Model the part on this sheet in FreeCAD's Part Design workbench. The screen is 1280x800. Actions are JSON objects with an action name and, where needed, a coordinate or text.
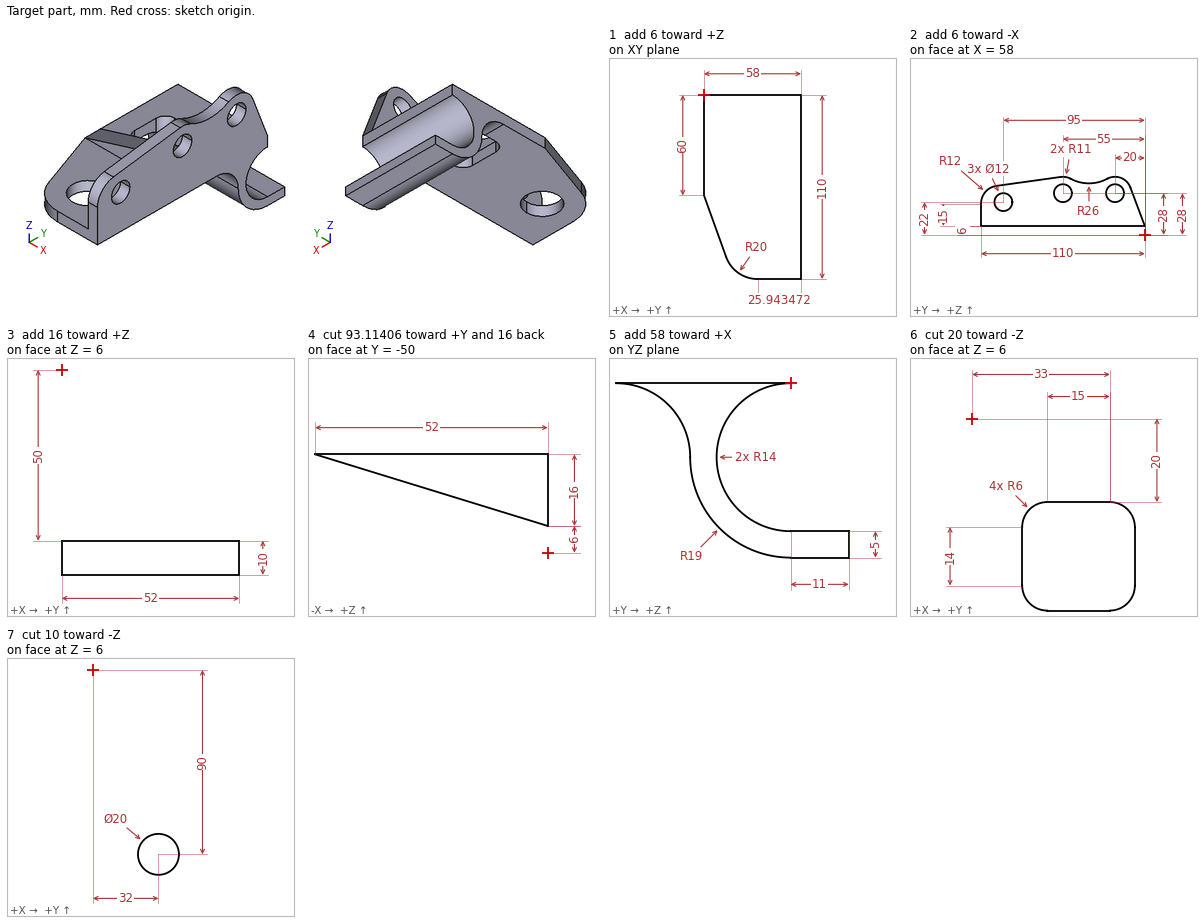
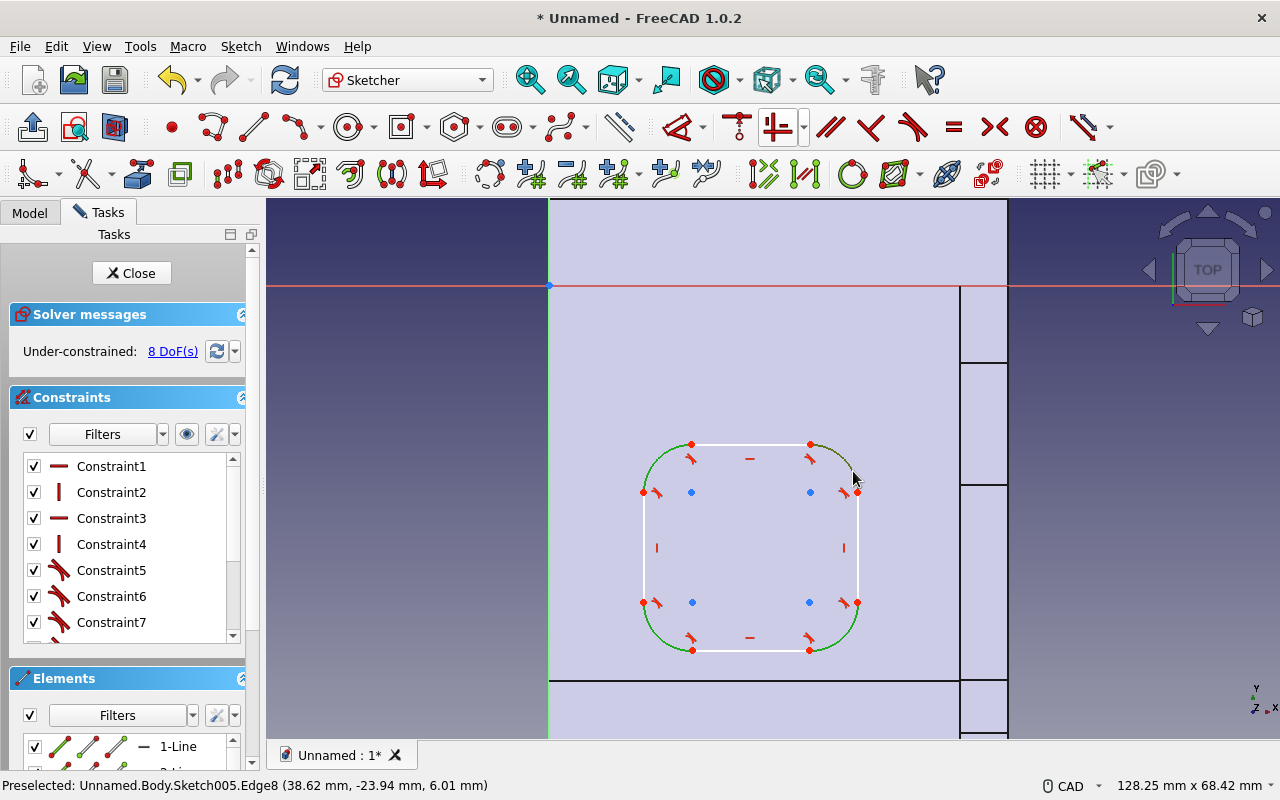
{"action": "left_click", "coordinate": [954, 128]}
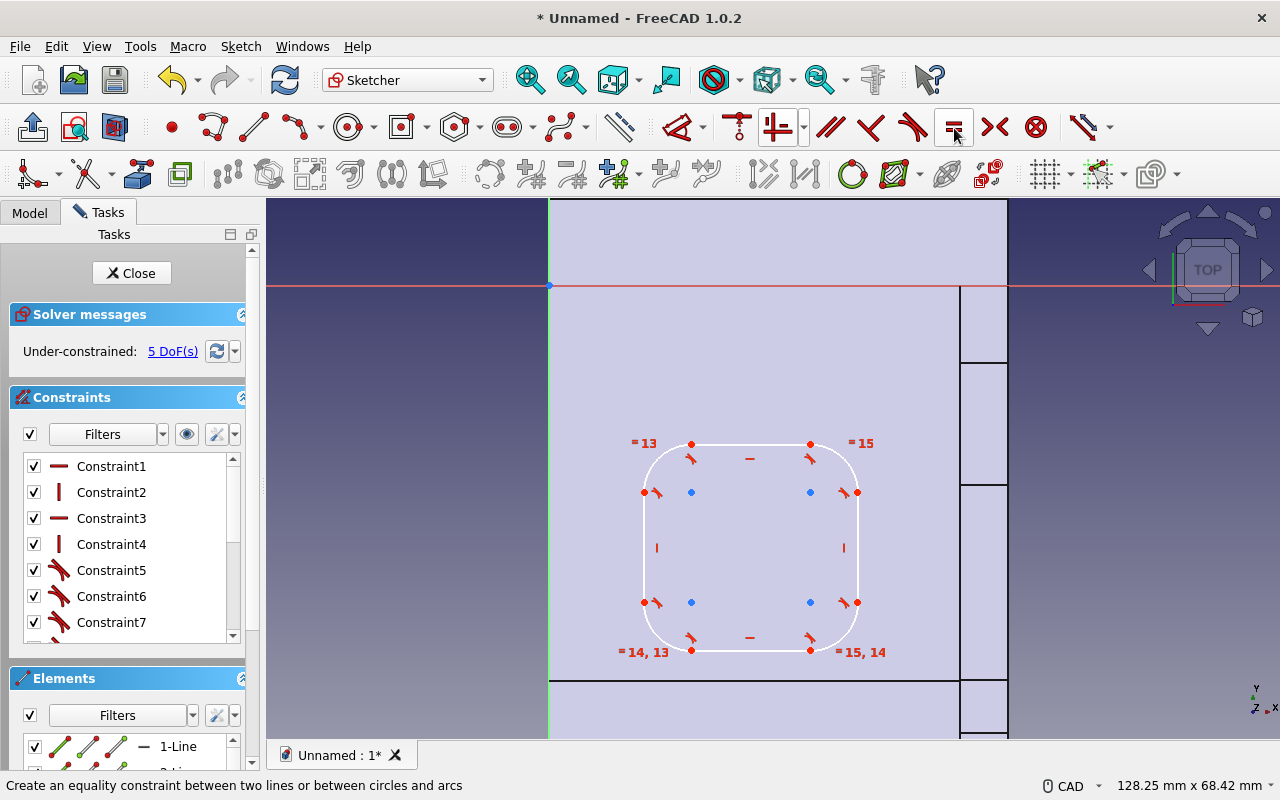
{"action": "key", "text": "d"}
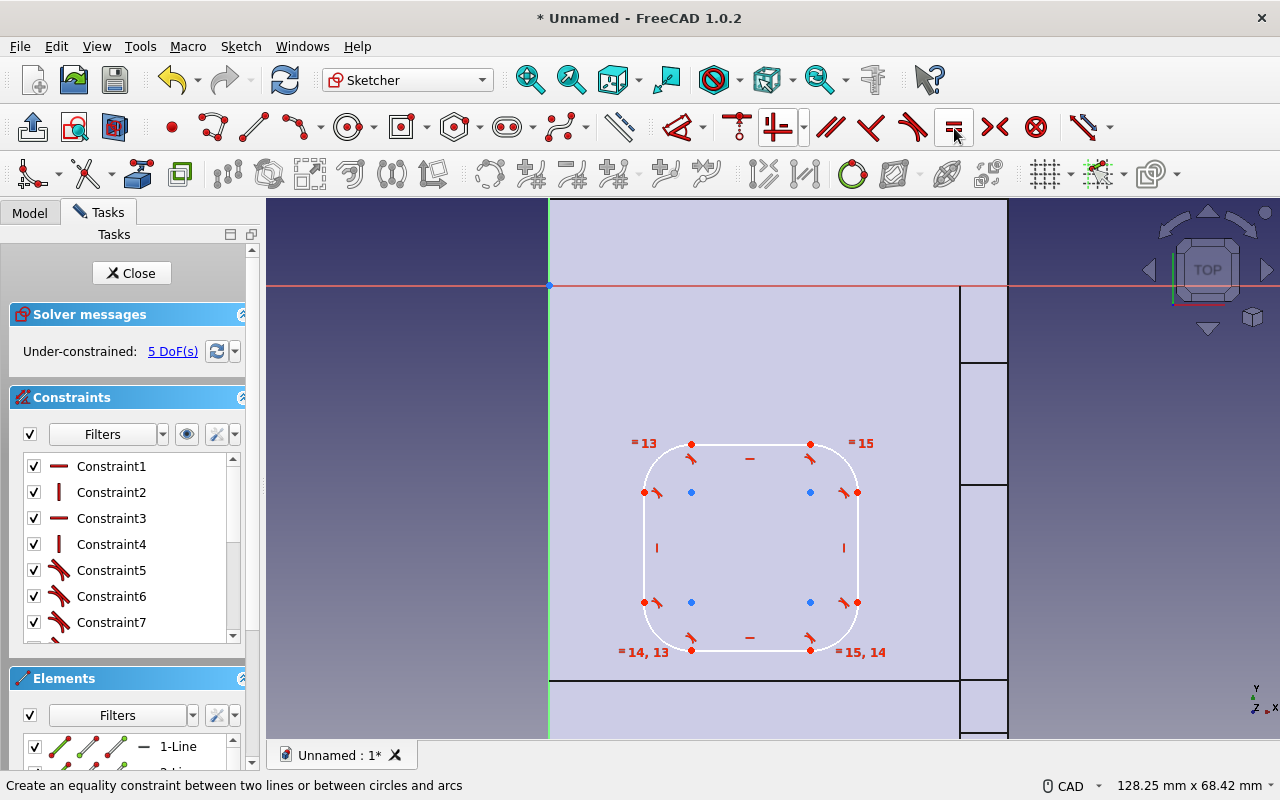
{"action": "left_click", "coordinate": [670, 450]}
{"action": "left_click", "coordinate": [655, 422]}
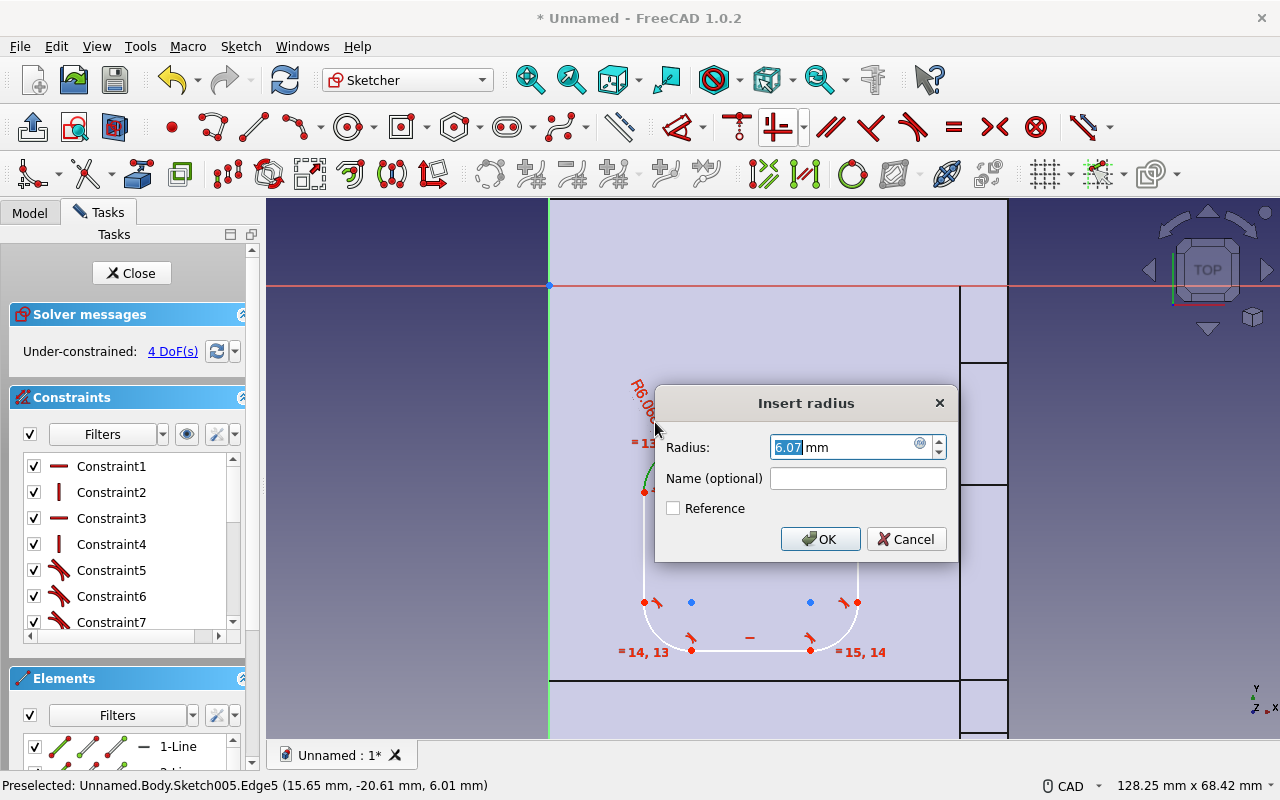
{"action": "type", "text": "6"}
{"action": "key", "text": "Return"}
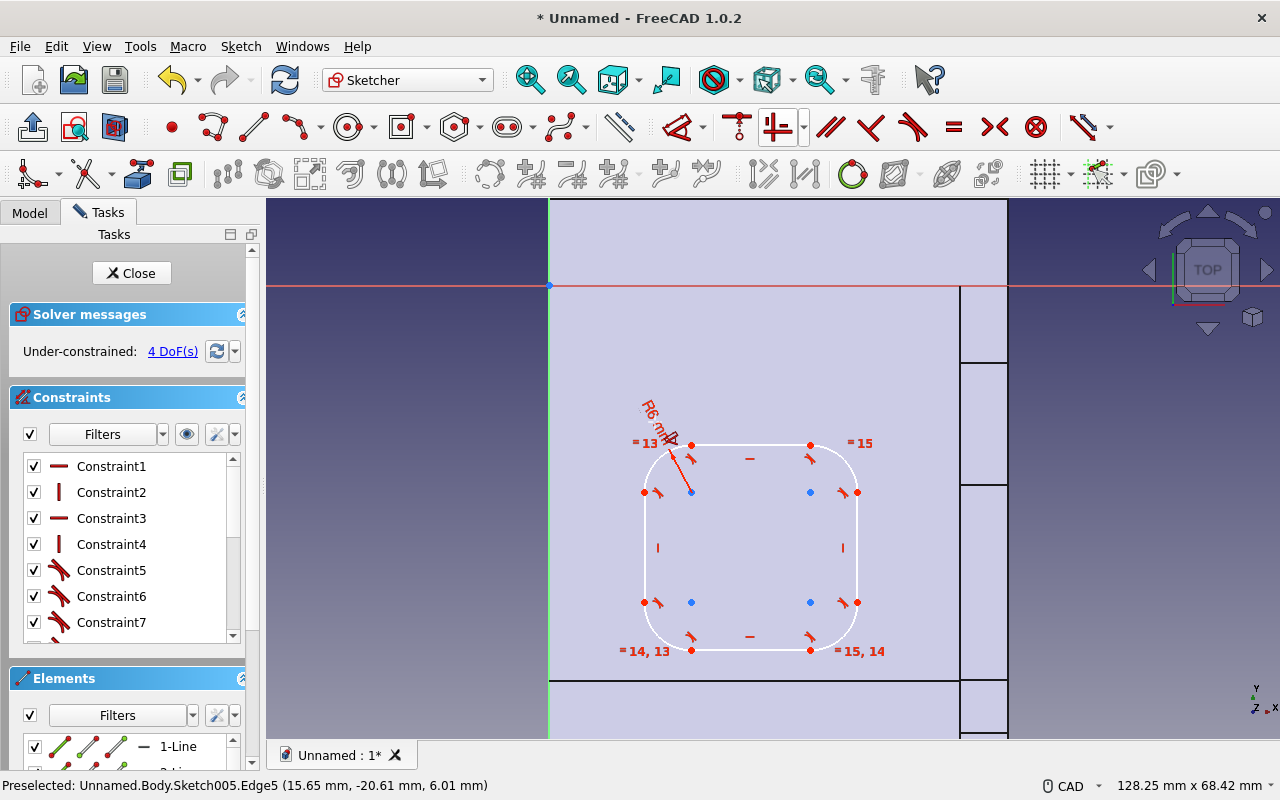
{"action": "left_click", "coordinate": [775, 445]}
{"action": "left_click", "coordinate": [751, 411]}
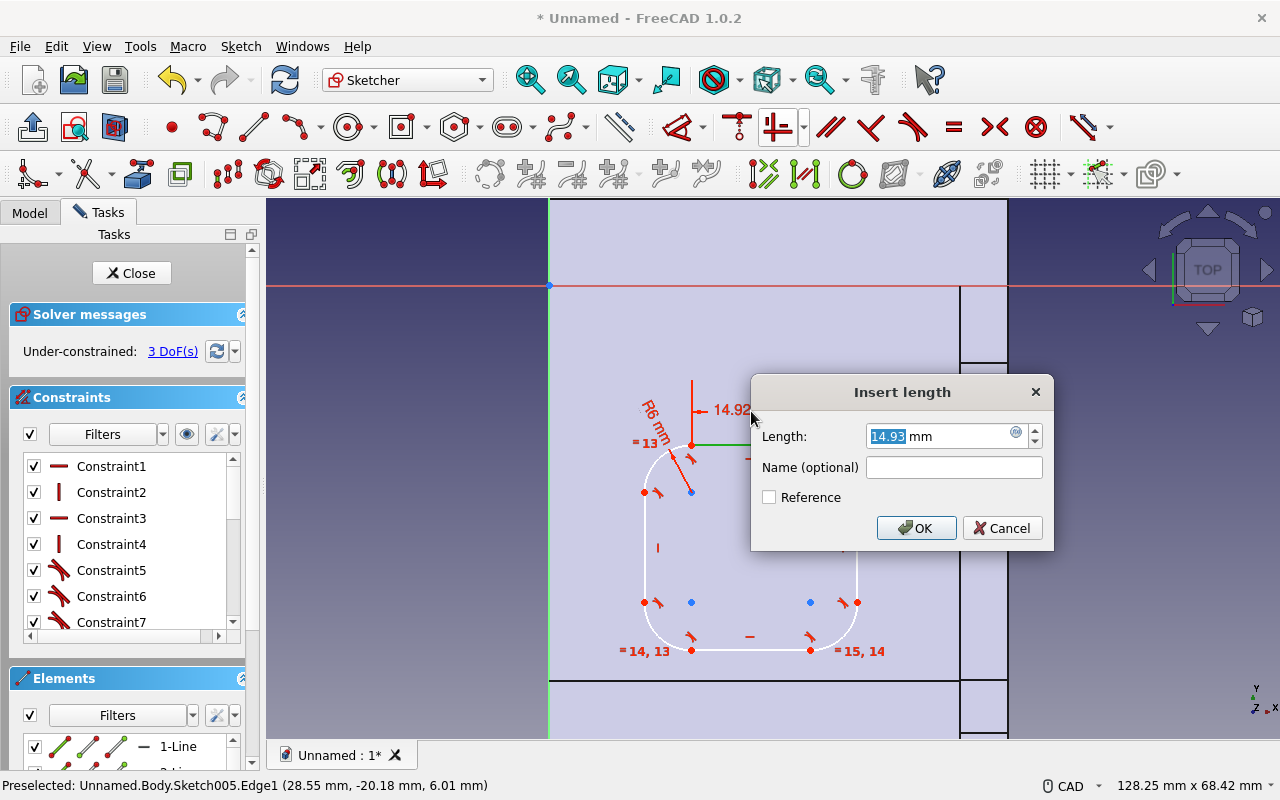
{"action": "type", "text": "15"}
{"action": "key", "text": "Return"}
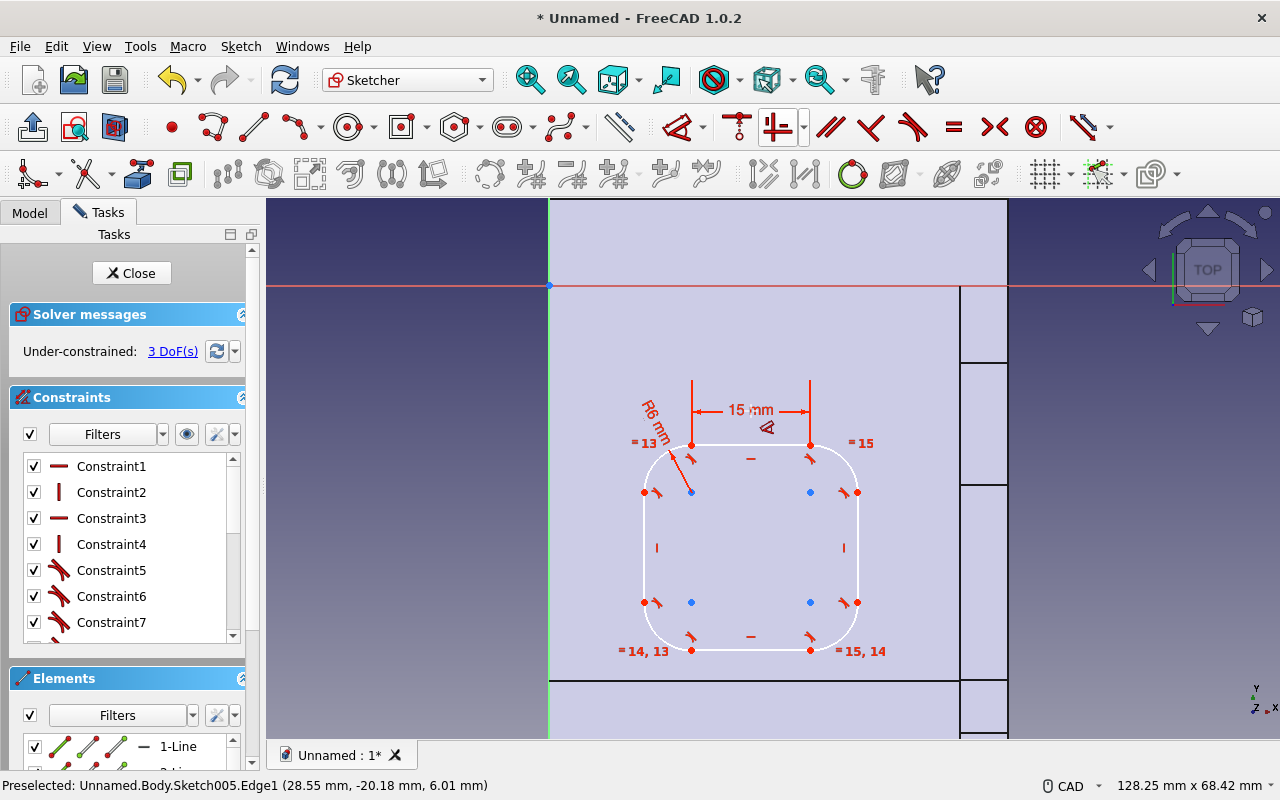
{"action": "left_click", "coordinate": [644, 526]}
{"action": "left_click", "coordinate": [610, 548]}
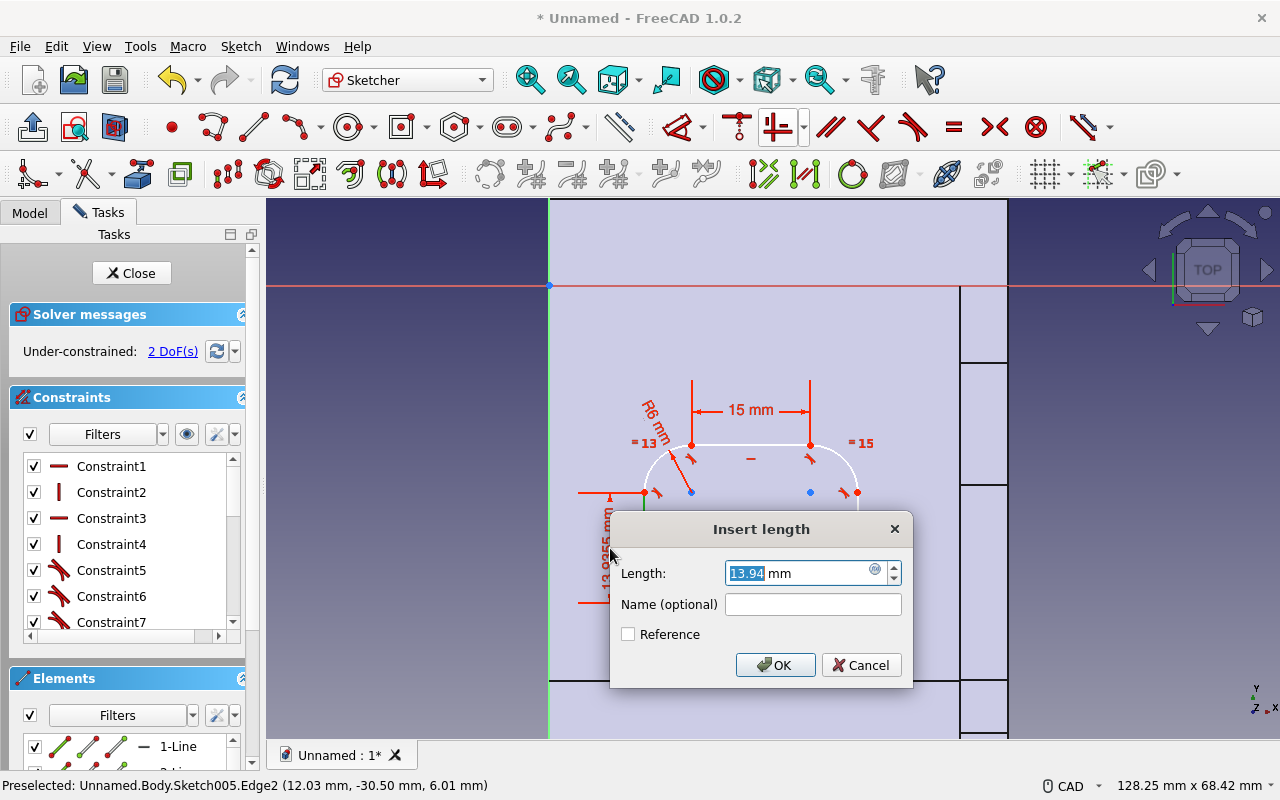
{"action": "type", "text": "14"}
{"action": "key", "text": "Return"}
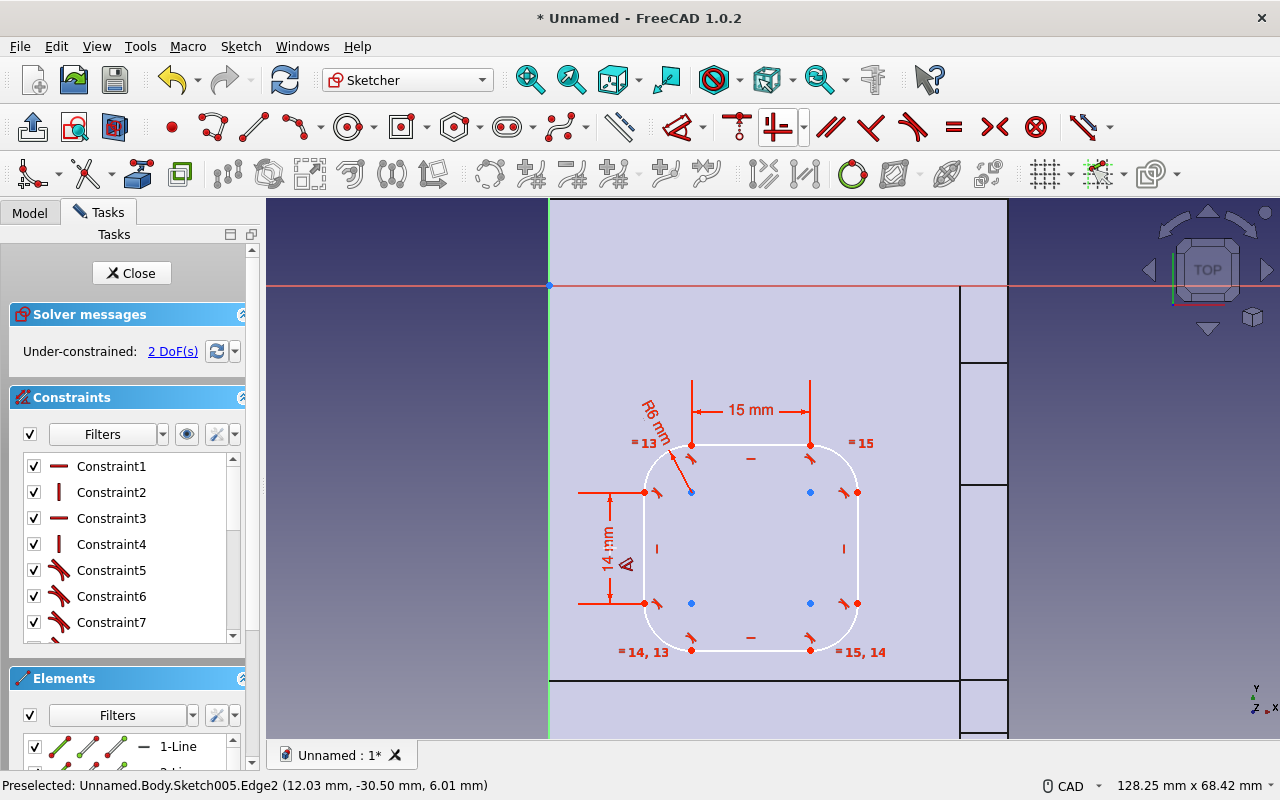
{"action": "left_click", "coordinate": [810, 445]}
{"action": "left_click", "coordinate": [680, 252]}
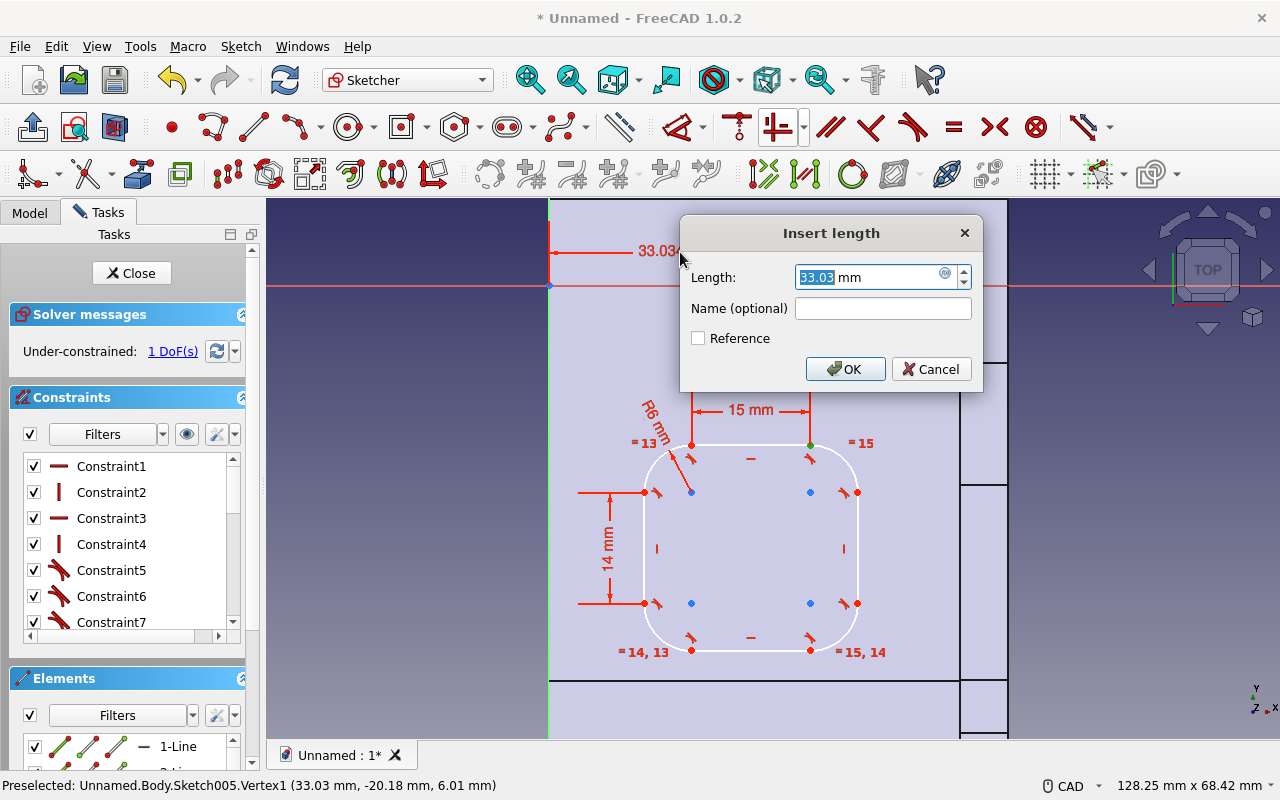
{"action": "type", "text": "33"}
{"action": "key", "text": "Return"}